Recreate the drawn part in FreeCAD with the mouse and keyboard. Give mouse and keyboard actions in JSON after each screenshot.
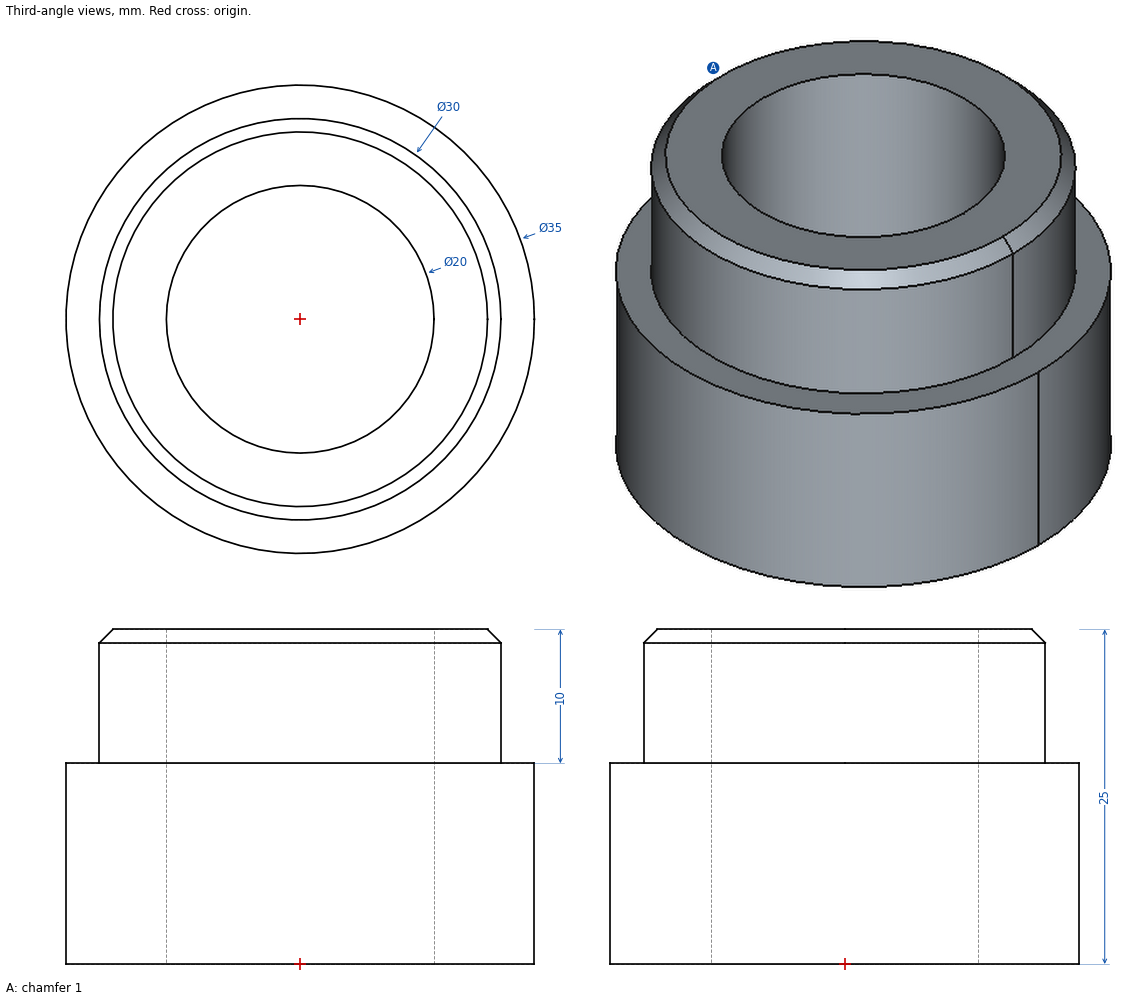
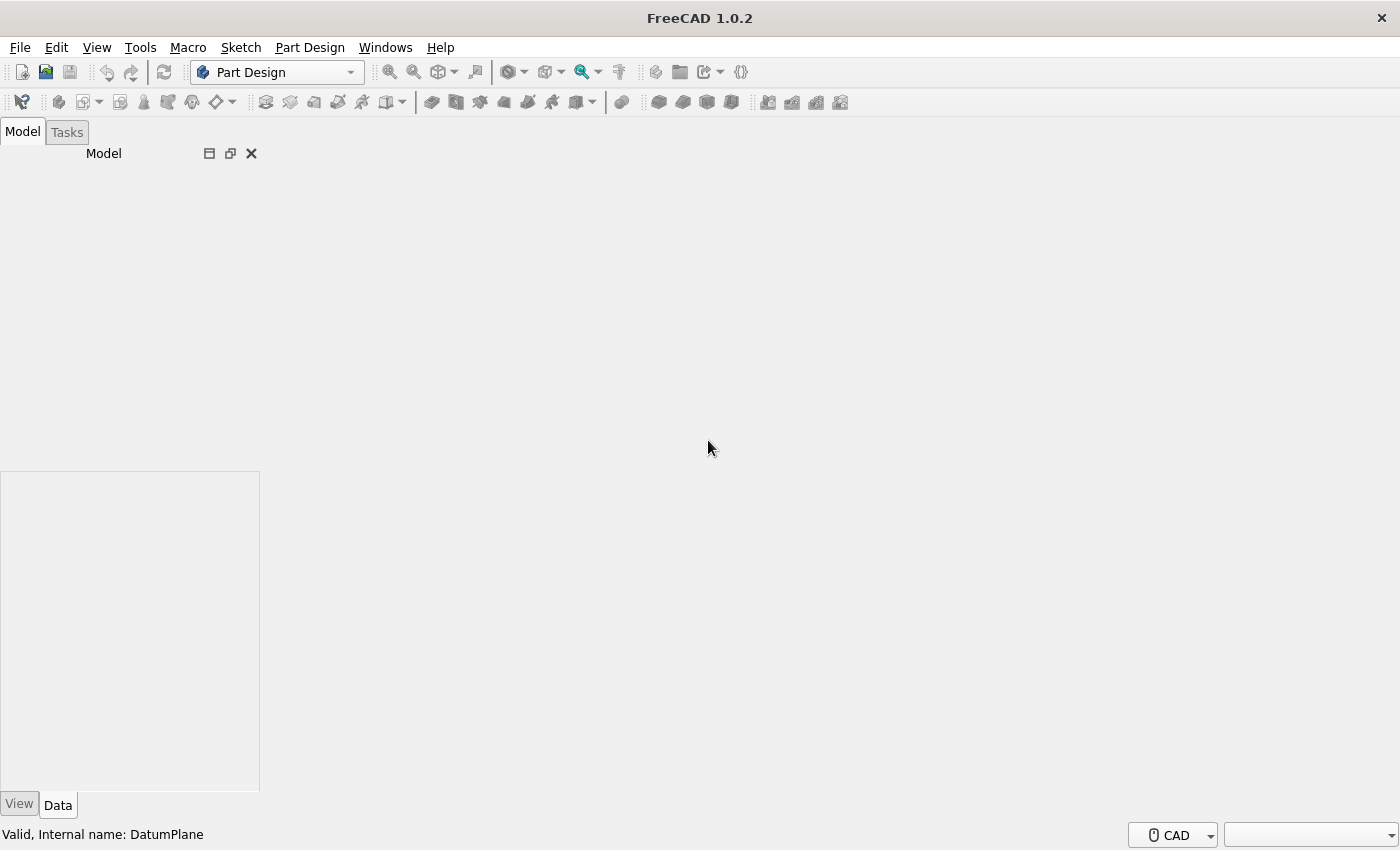
{"action": "left_click", "coordinate": [22, 72]}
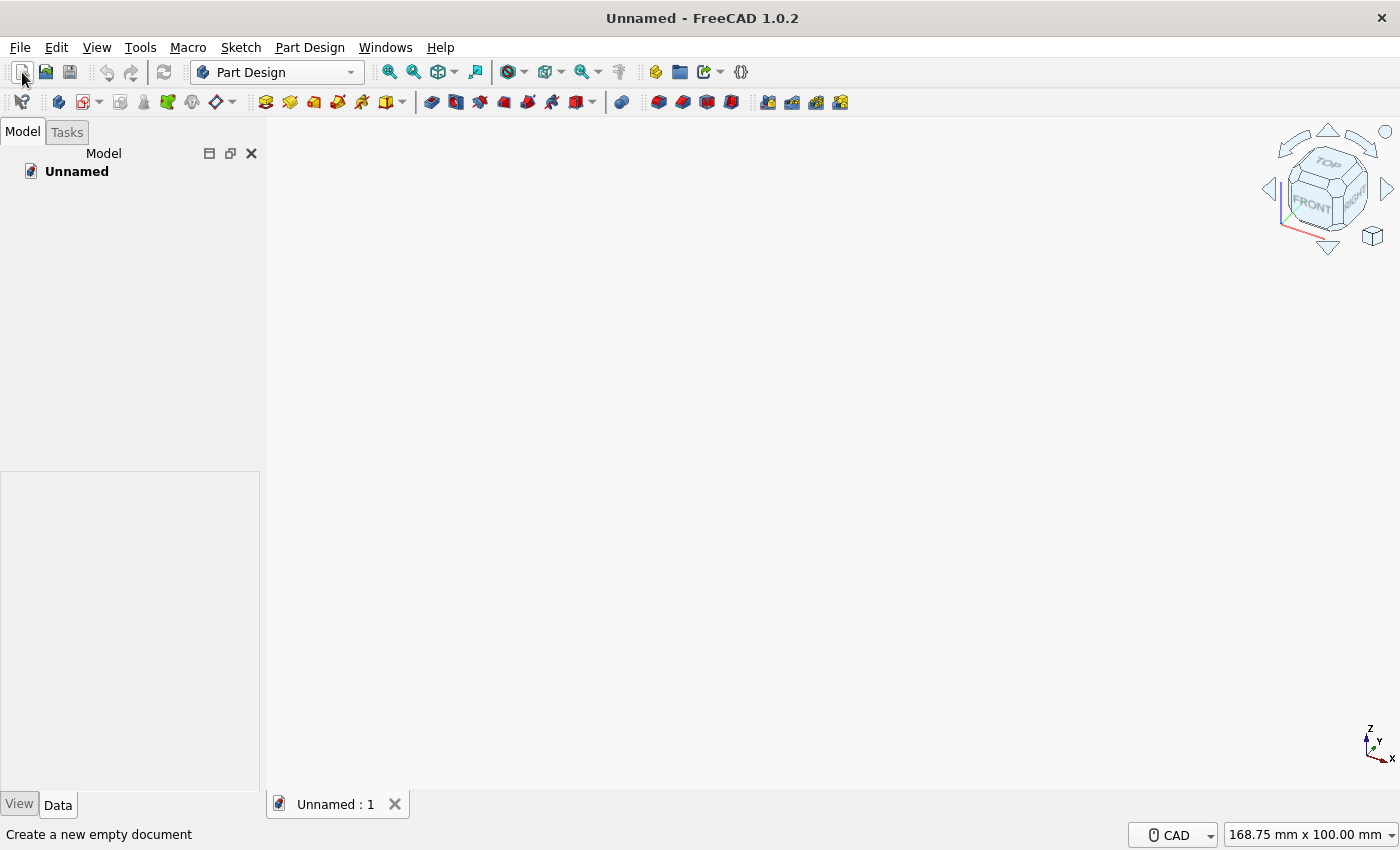
{"action": "left_click", "coordinate": [84, 102]}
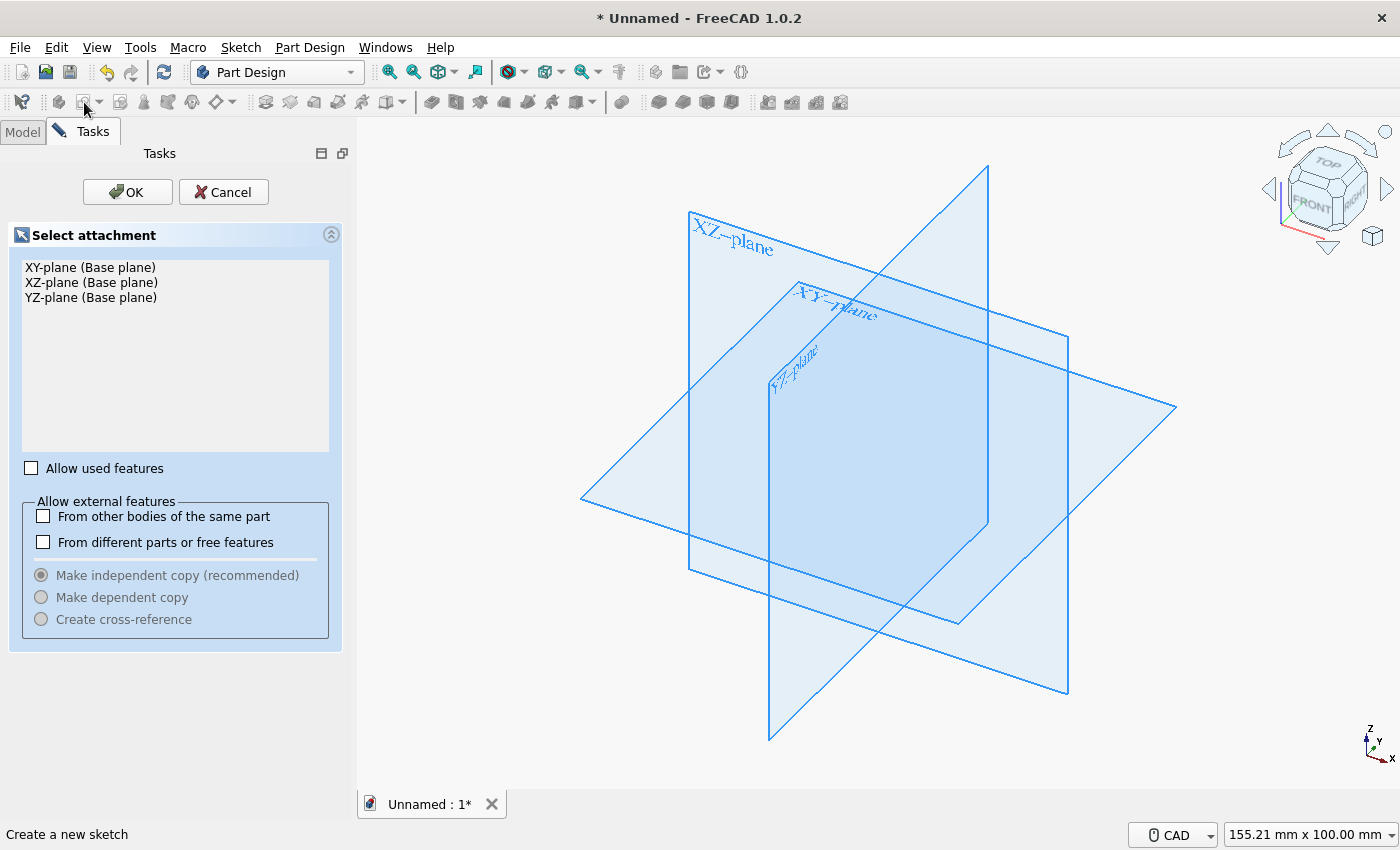
{"action": "left_click", "coordinate": [82, 268]}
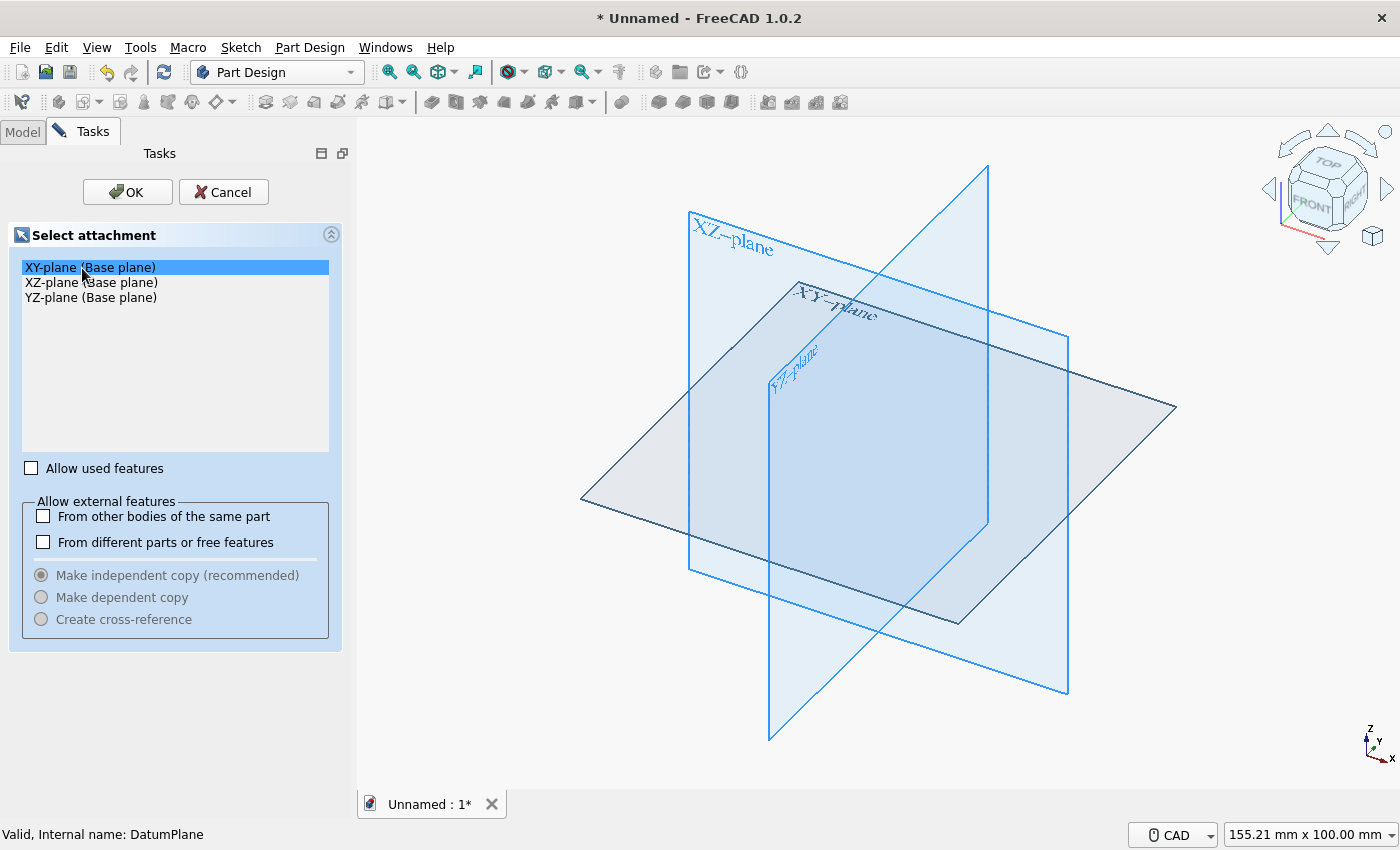
{"action": "left_click", "coordinate": [128, 192]}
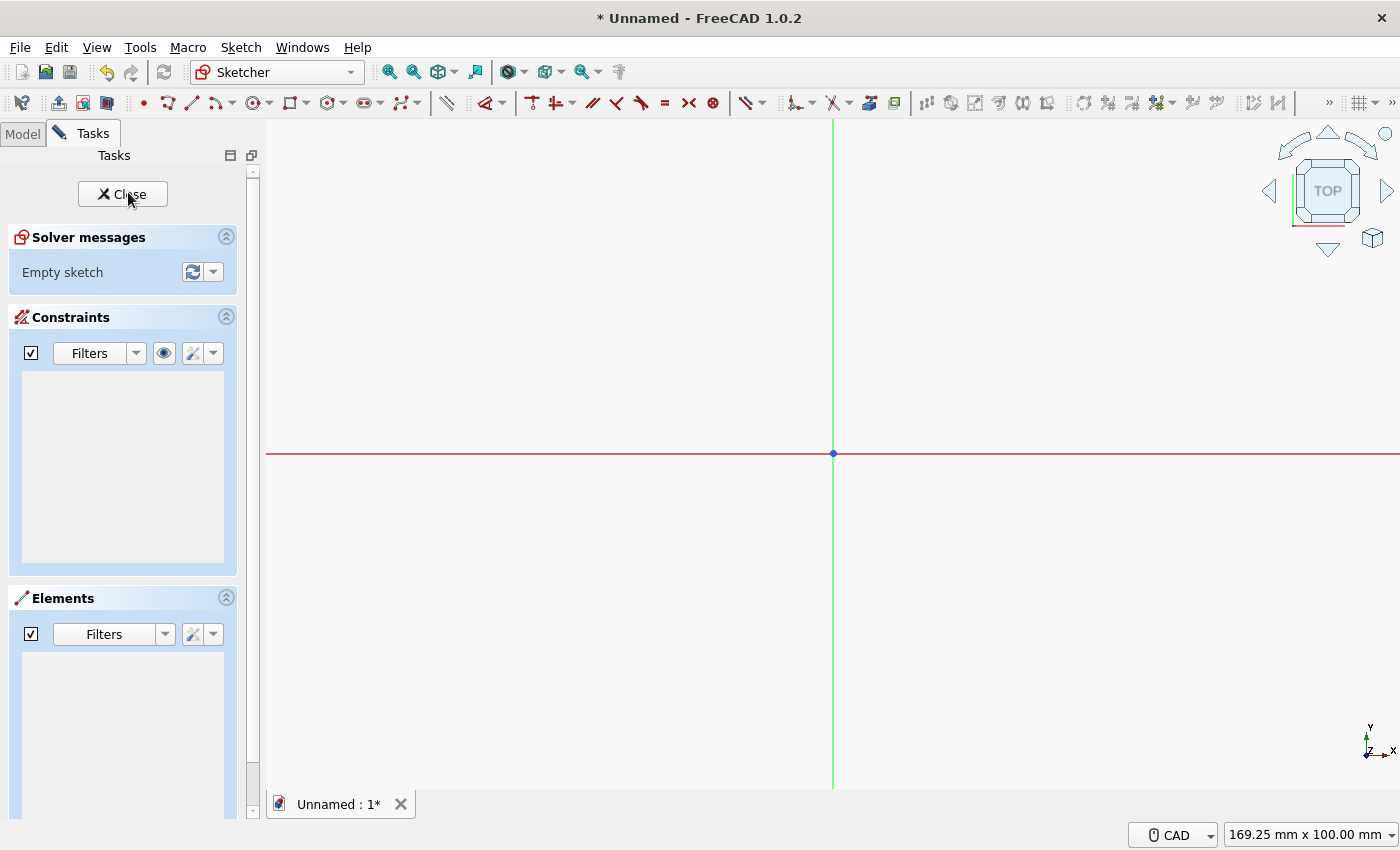
{"action": "scroll", "coordinate": [916, 454], "scroll_direction": "up", "scroll_amount": 3}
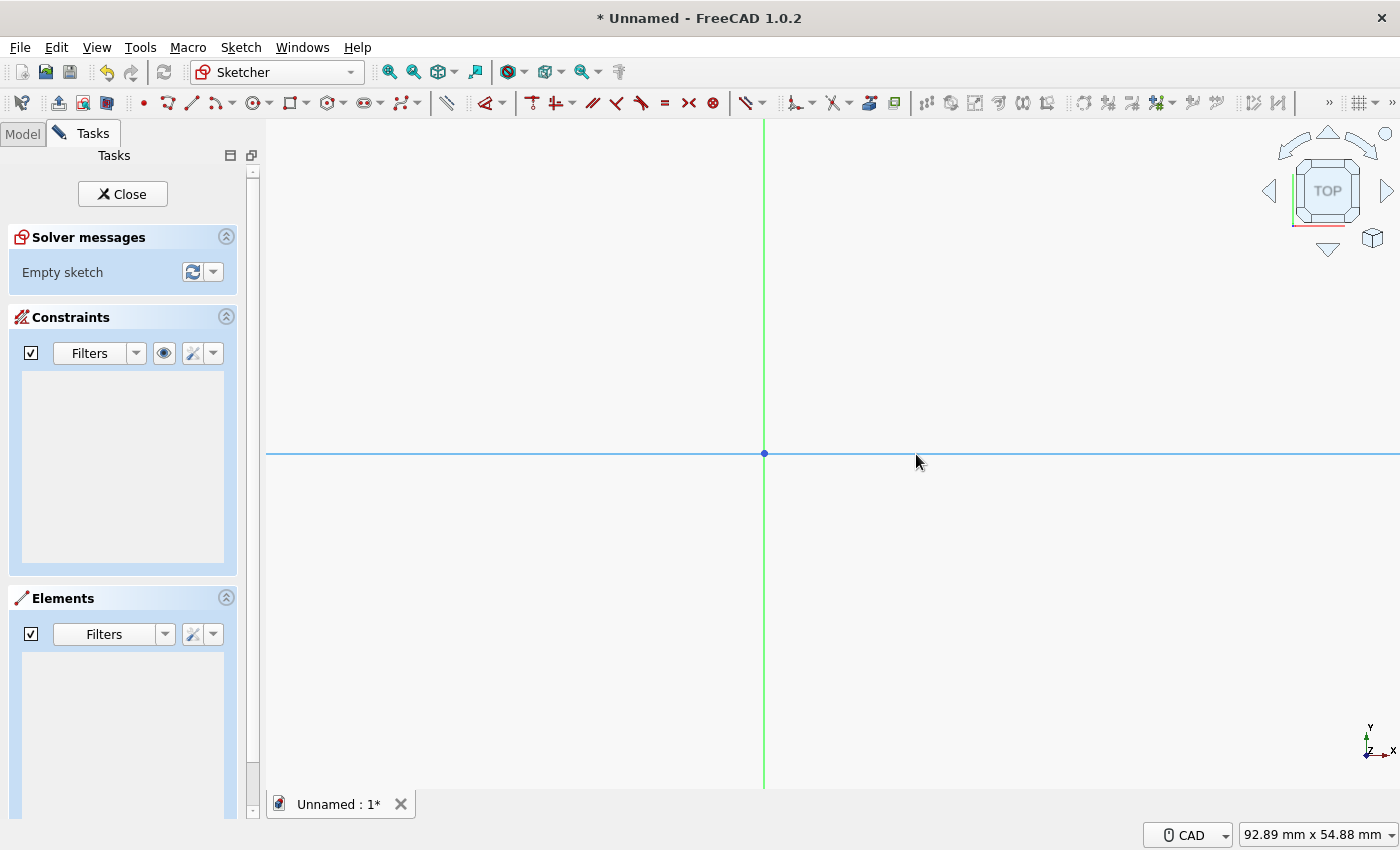
{"action": "left_click", "coordinate": [254, 104]}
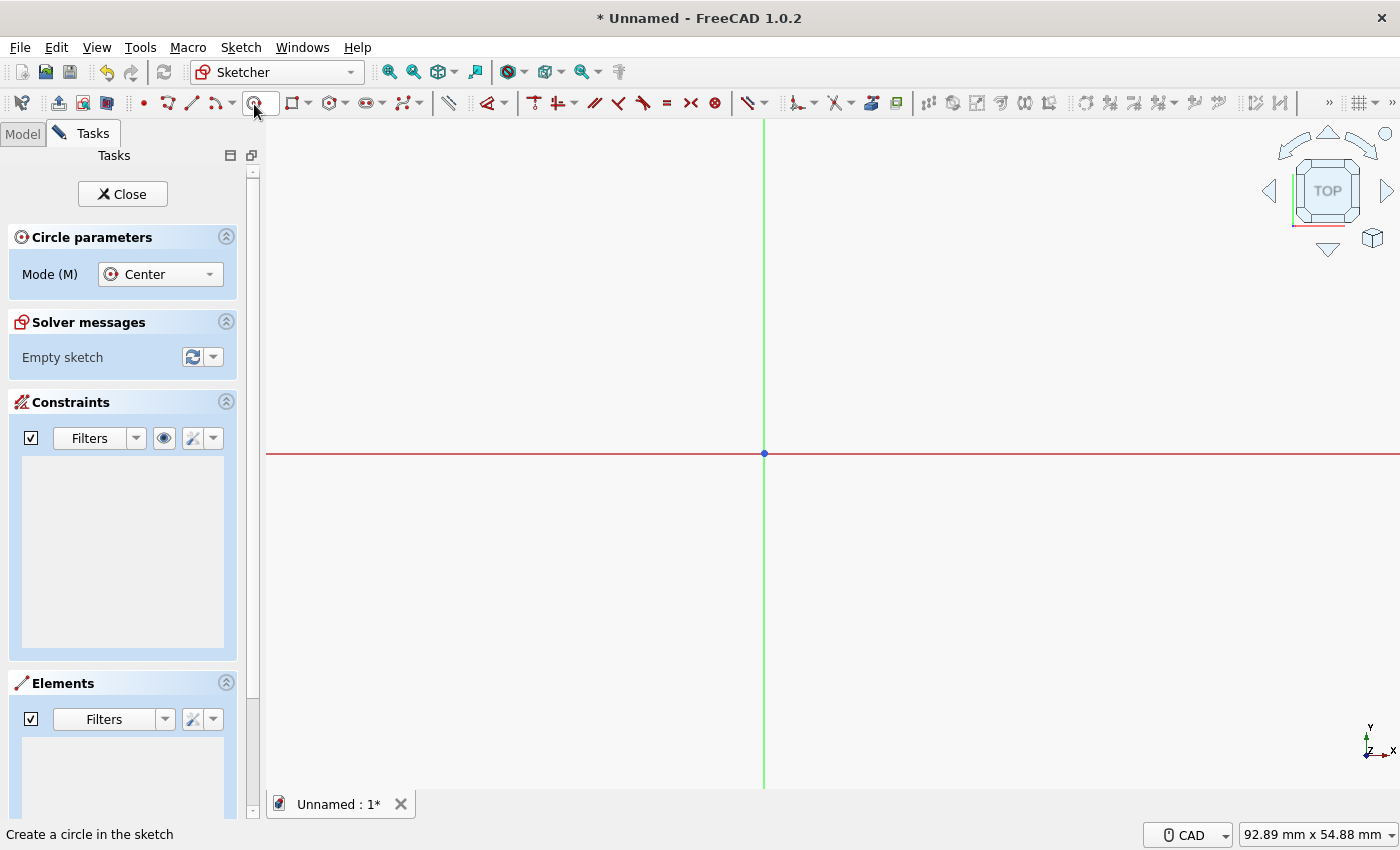
{"action": "left_click", "coordinate": [764, 454]}
{"action": "mouse_move", "coordinate": [915, 303]}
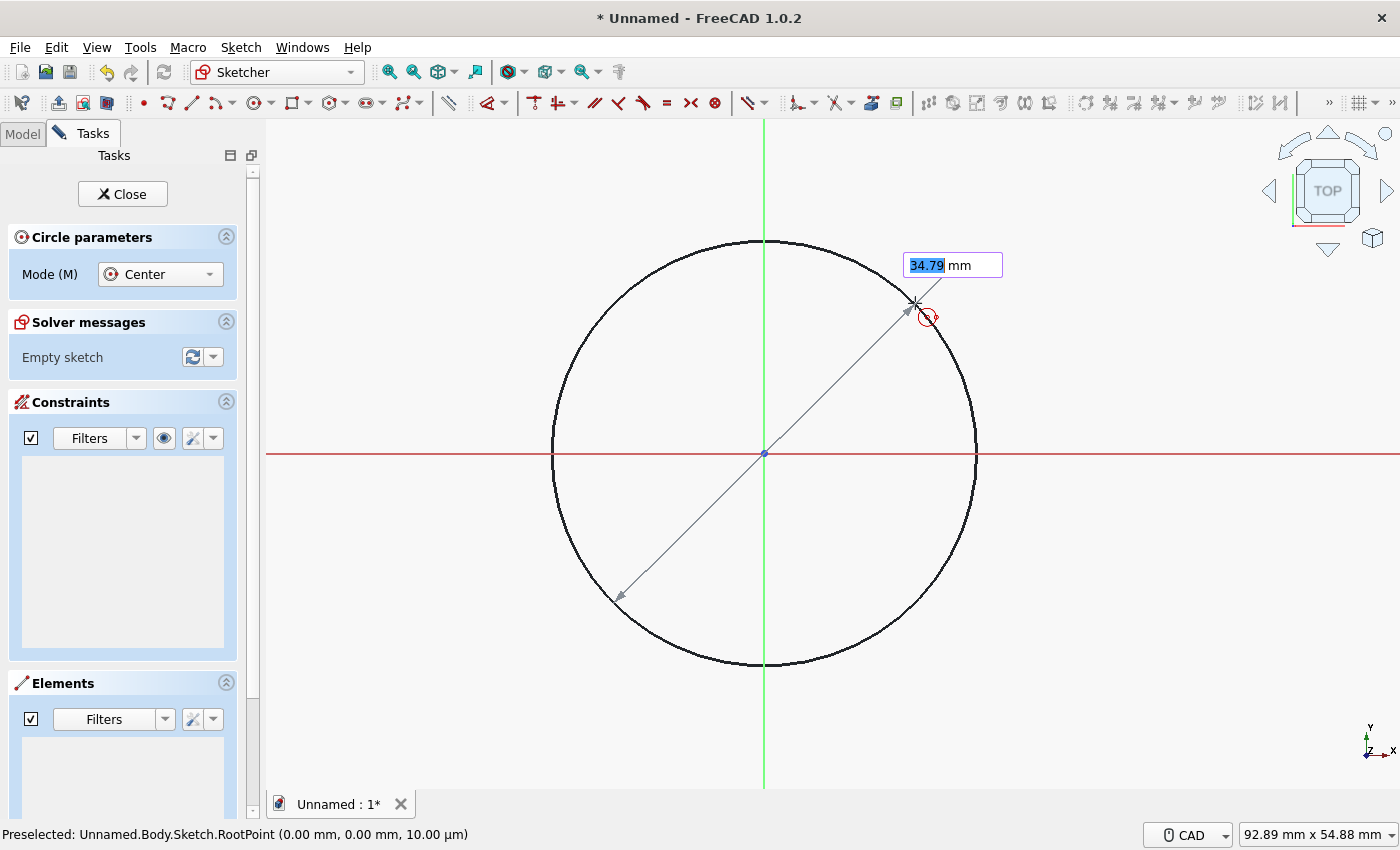
{"action": "type", "text": "35"}
{"action": "key", "text": "Return"}